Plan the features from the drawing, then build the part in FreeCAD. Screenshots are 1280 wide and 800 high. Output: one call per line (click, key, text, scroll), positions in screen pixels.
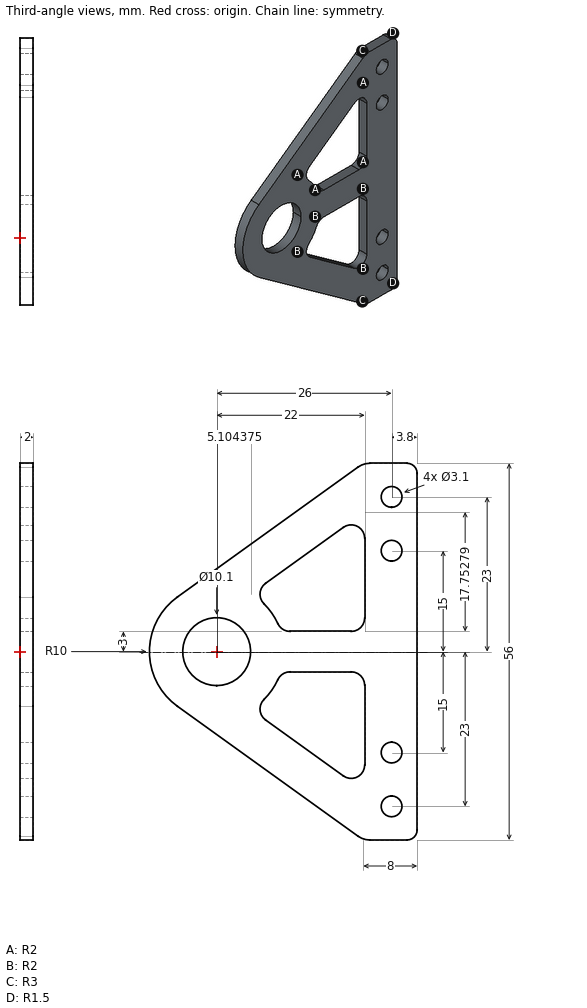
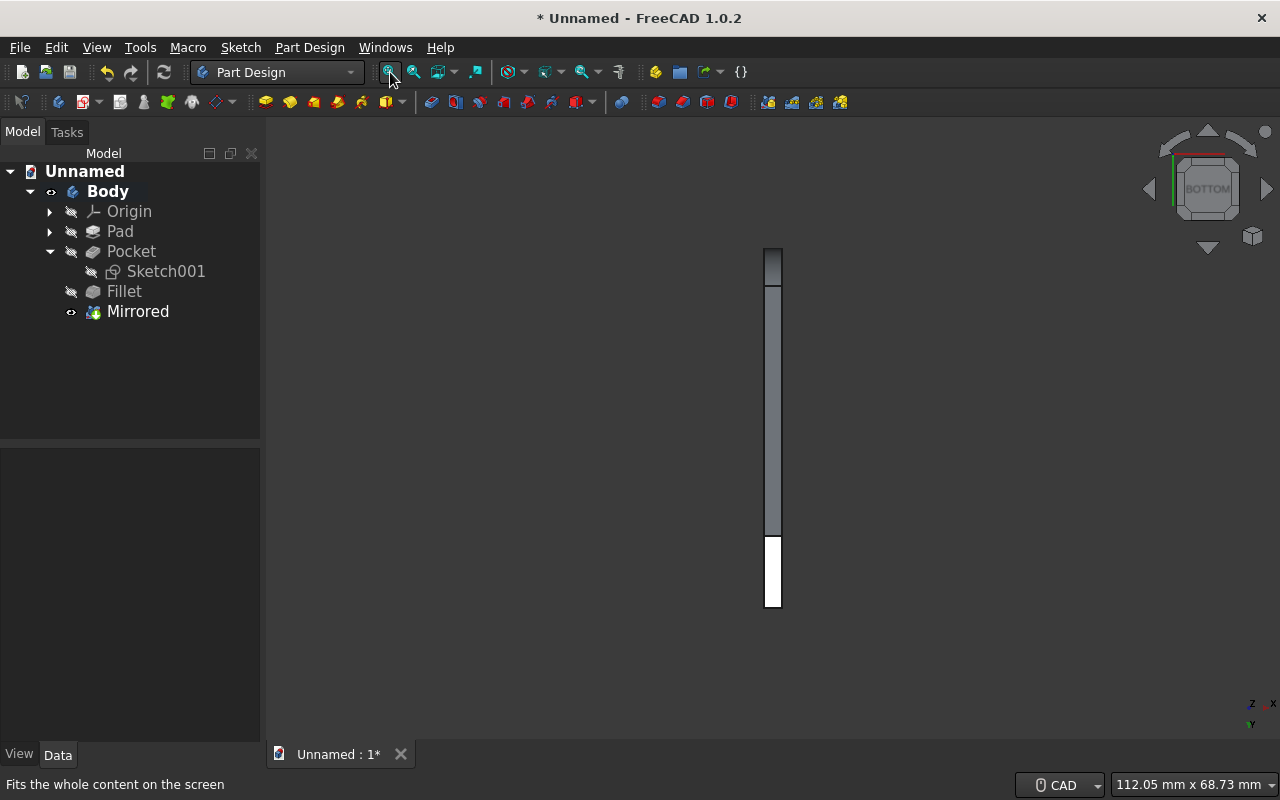
key(4)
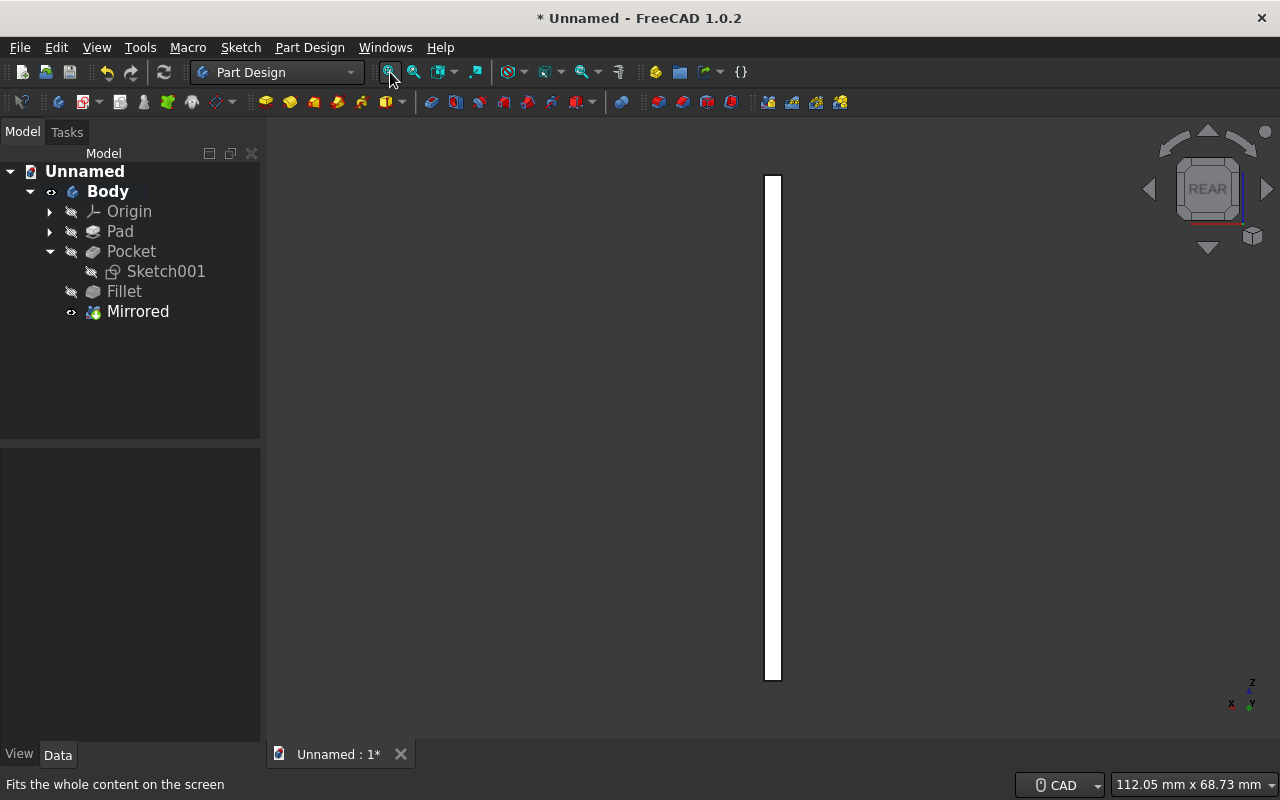
scroll(773, 615, up, 4)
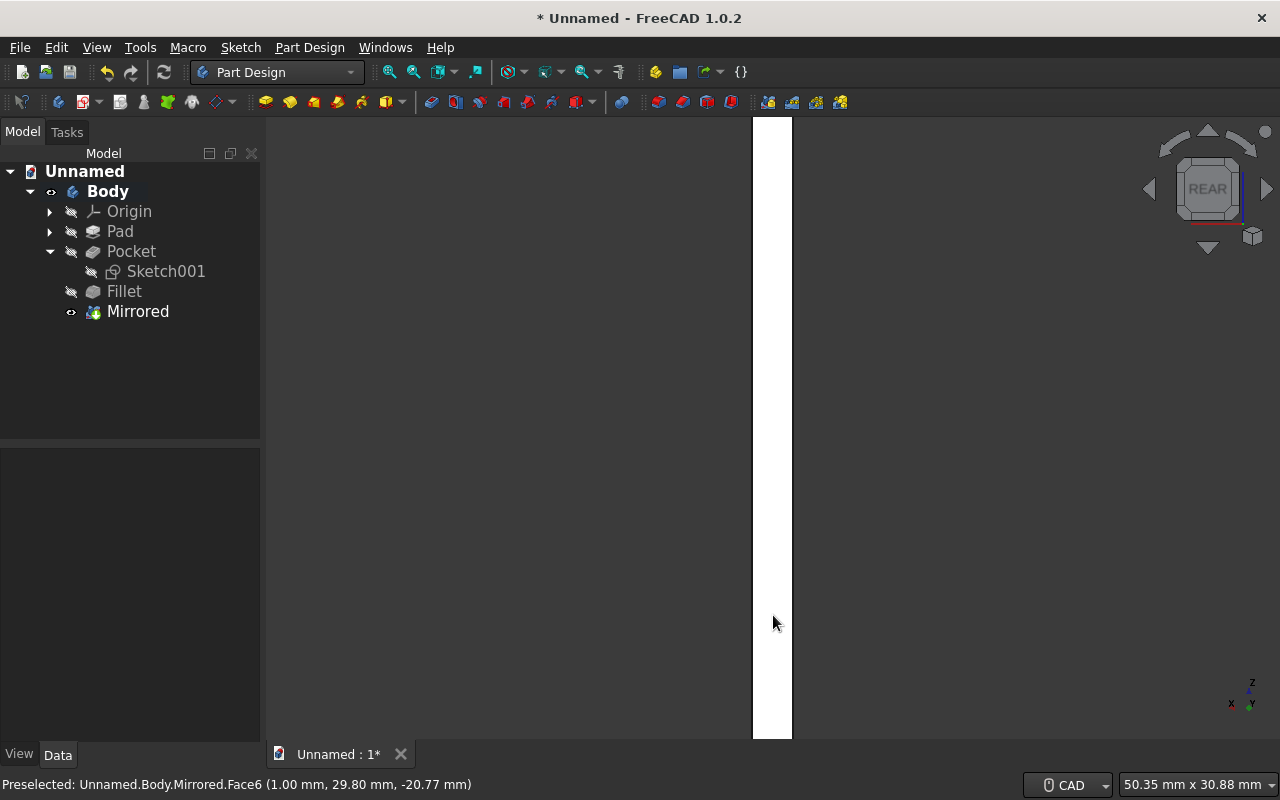
click(390, 72)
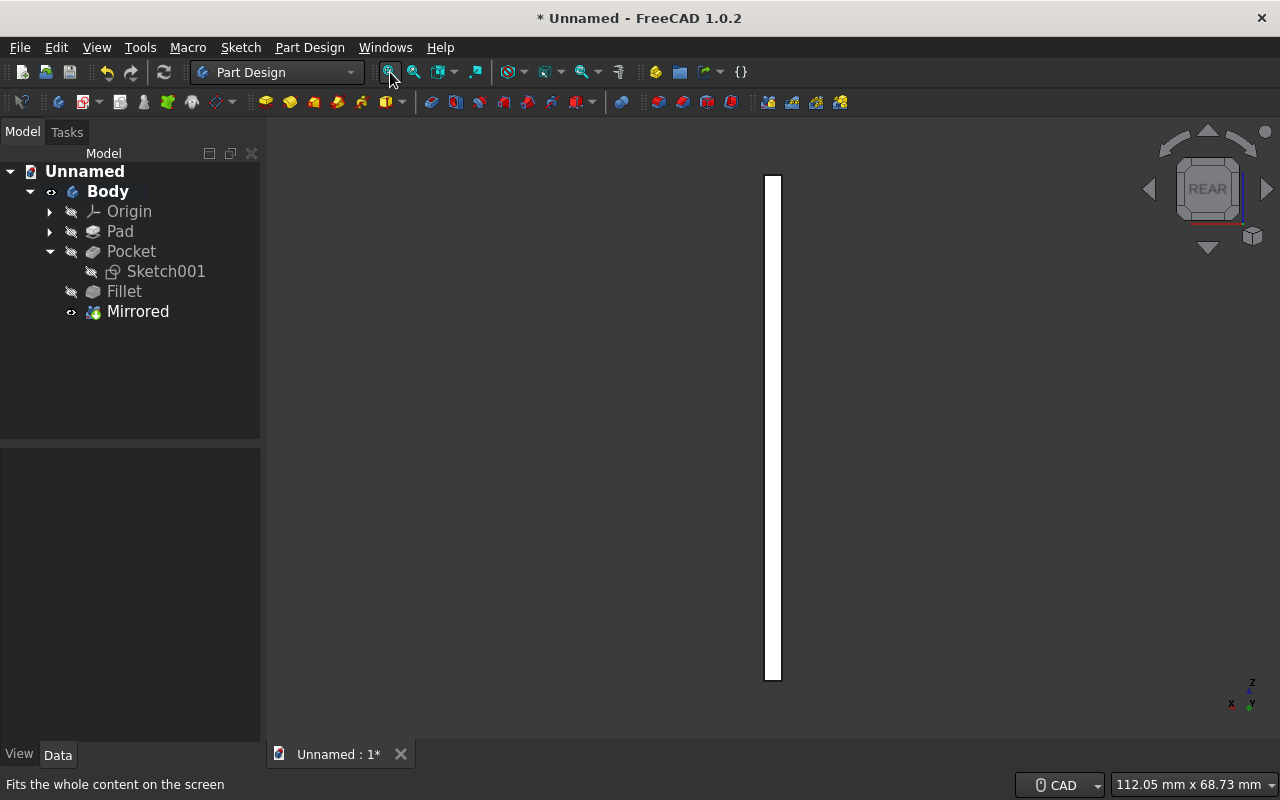
key(6)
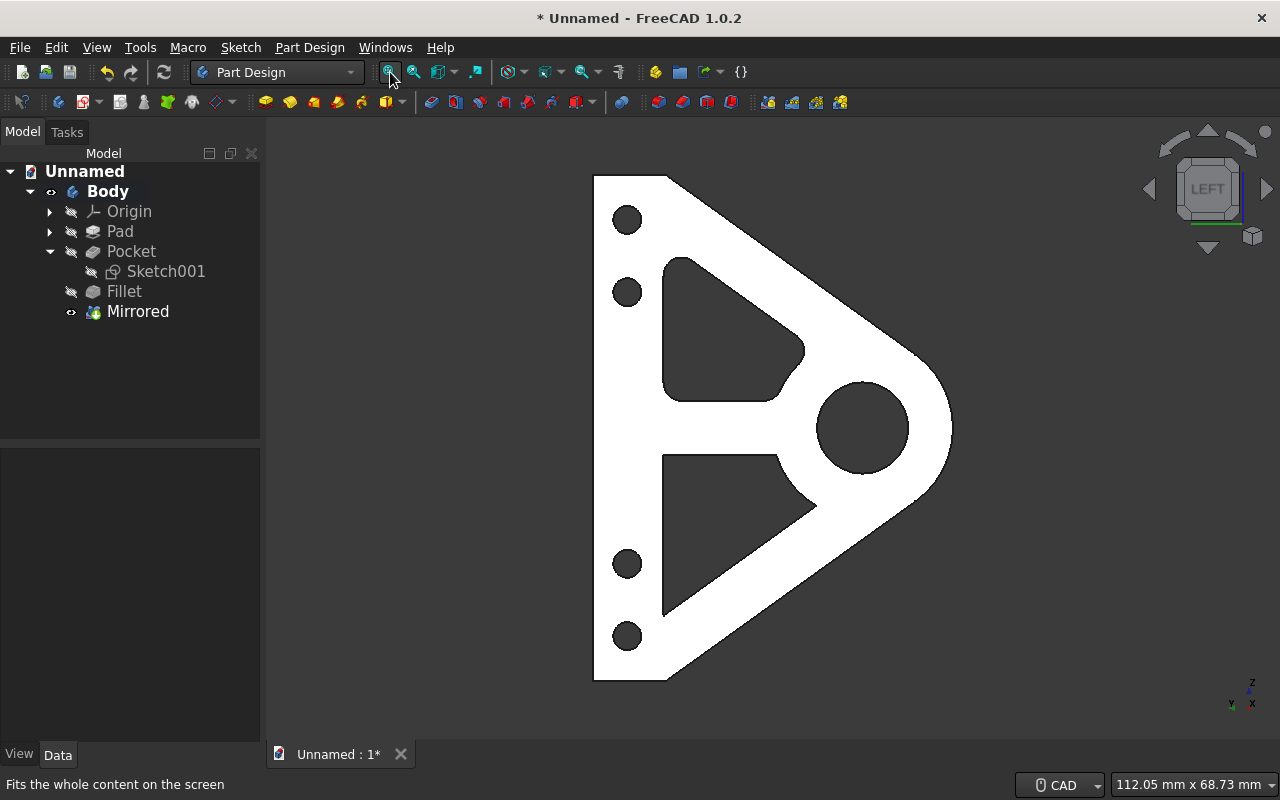
scroll(663, 615, up, 4)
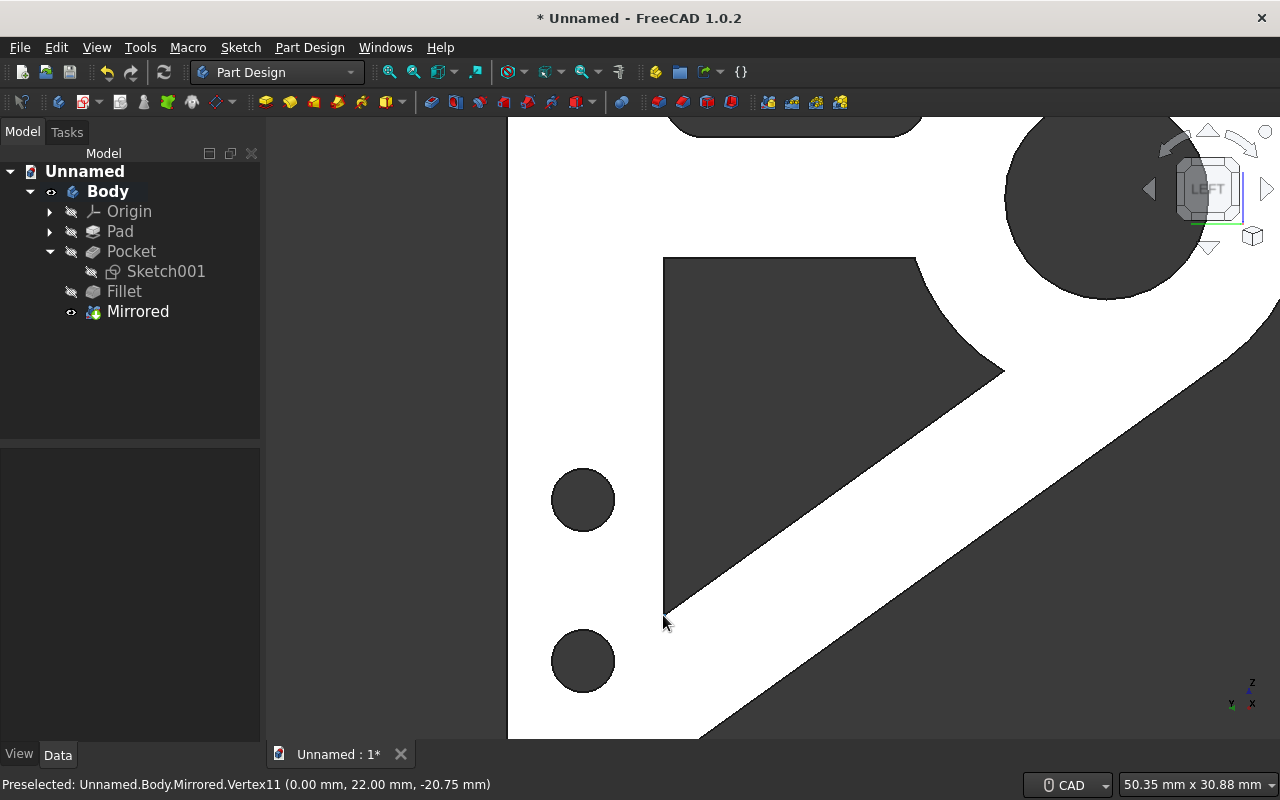
key(v)
key(f)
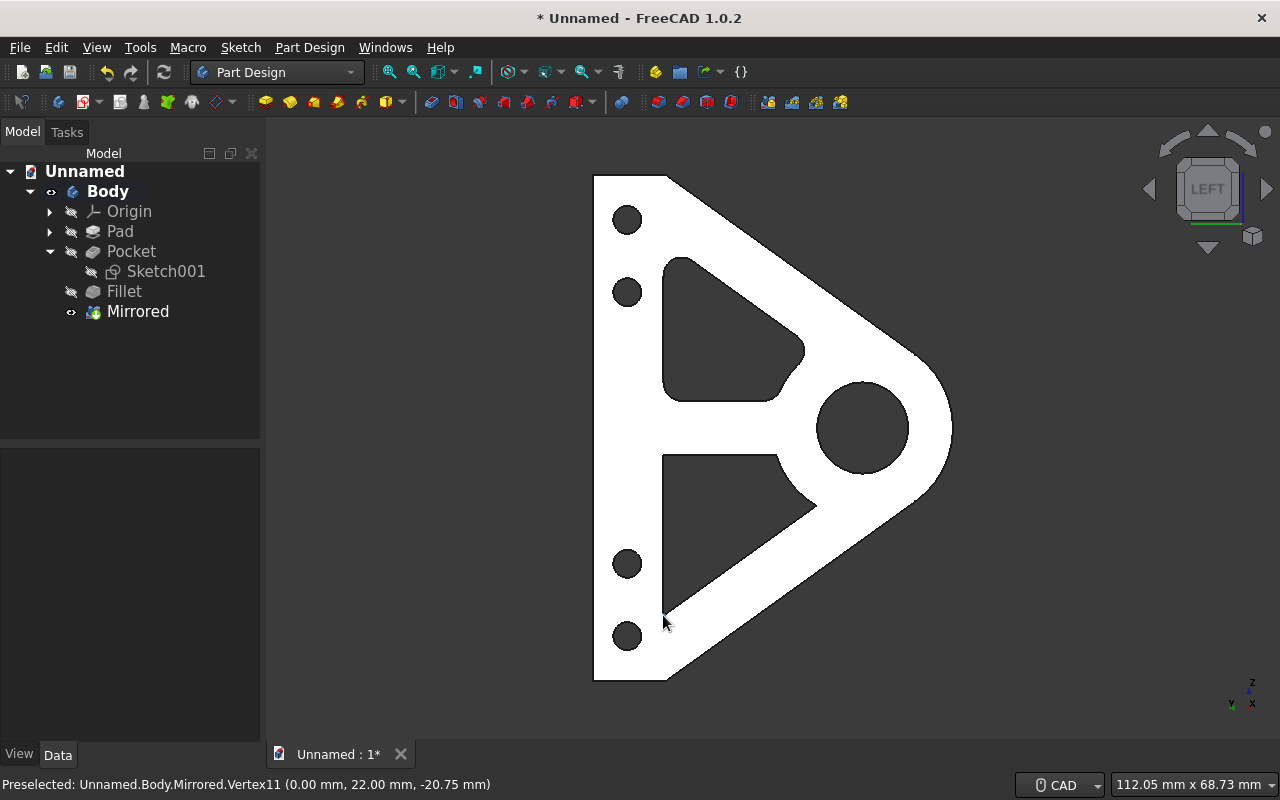
key(v)
key(3)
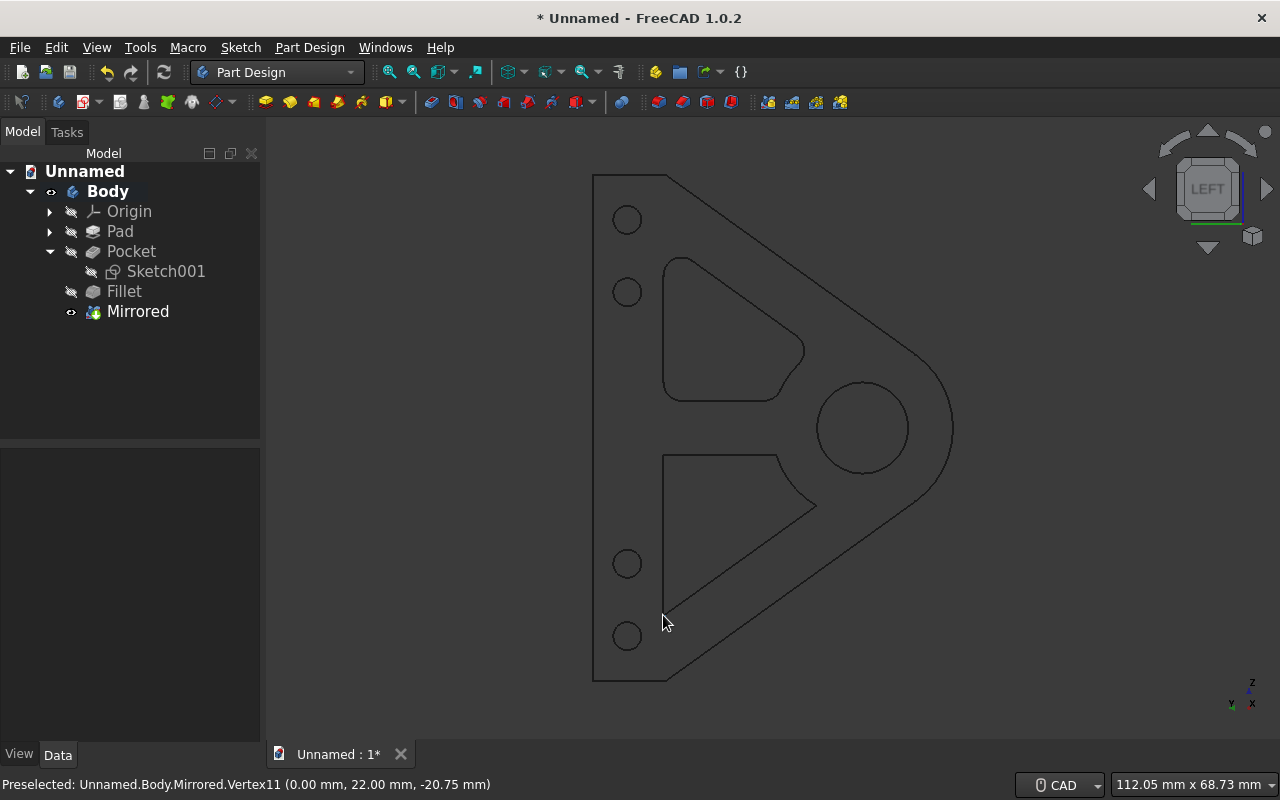
key(0)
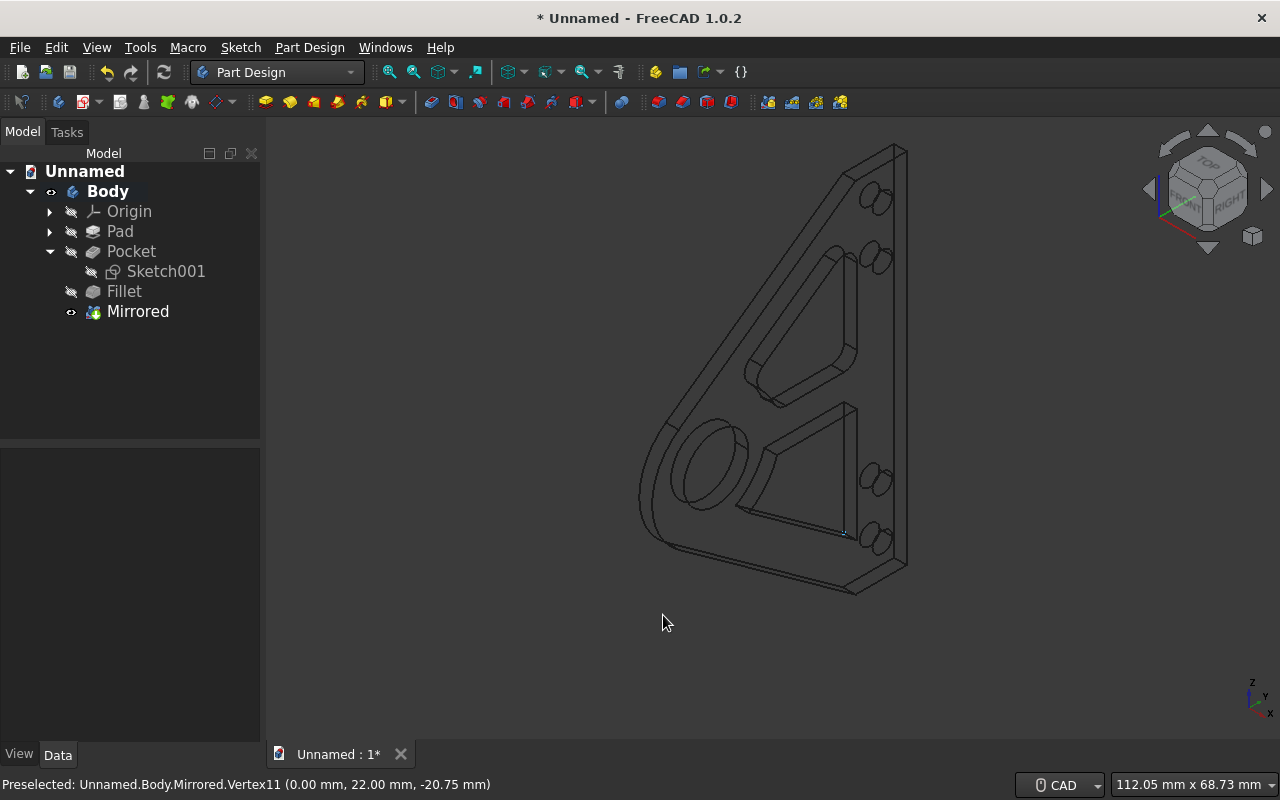
click(850, 404)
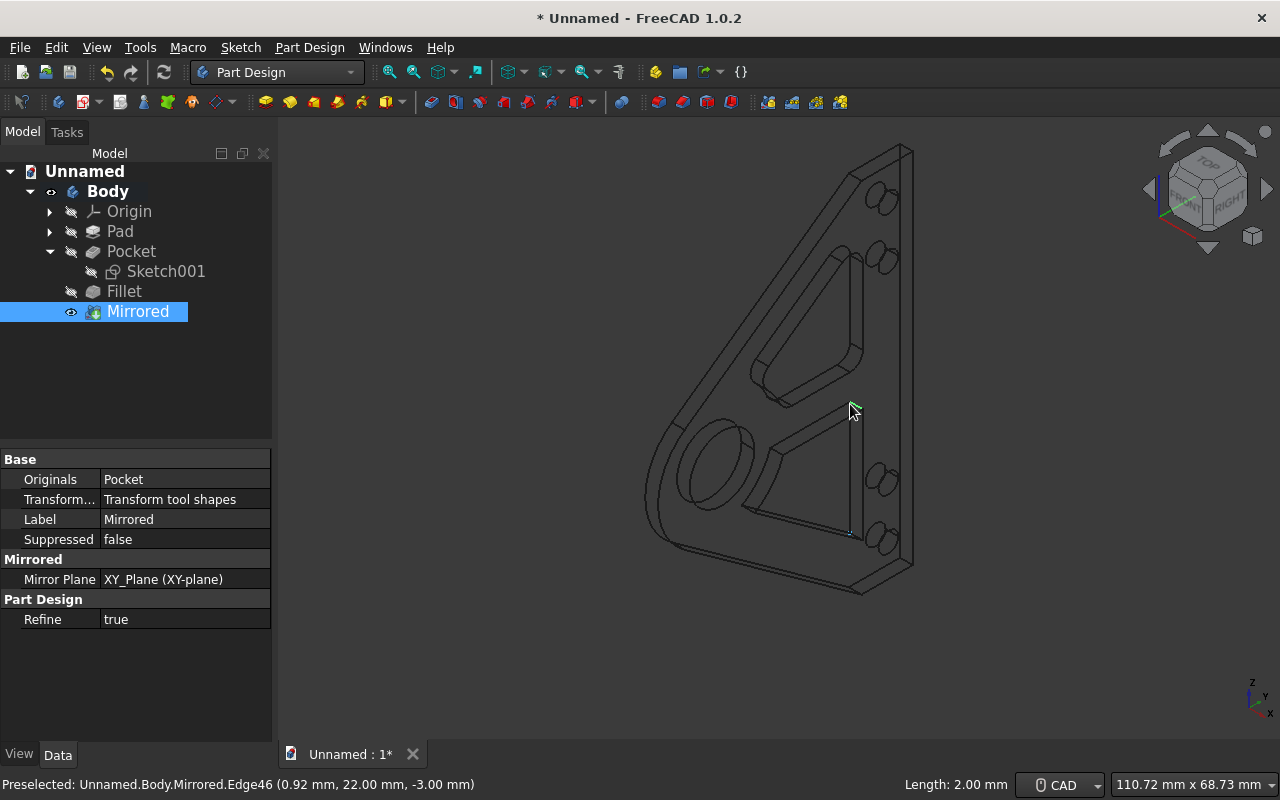
click(777, 450, ctrl)